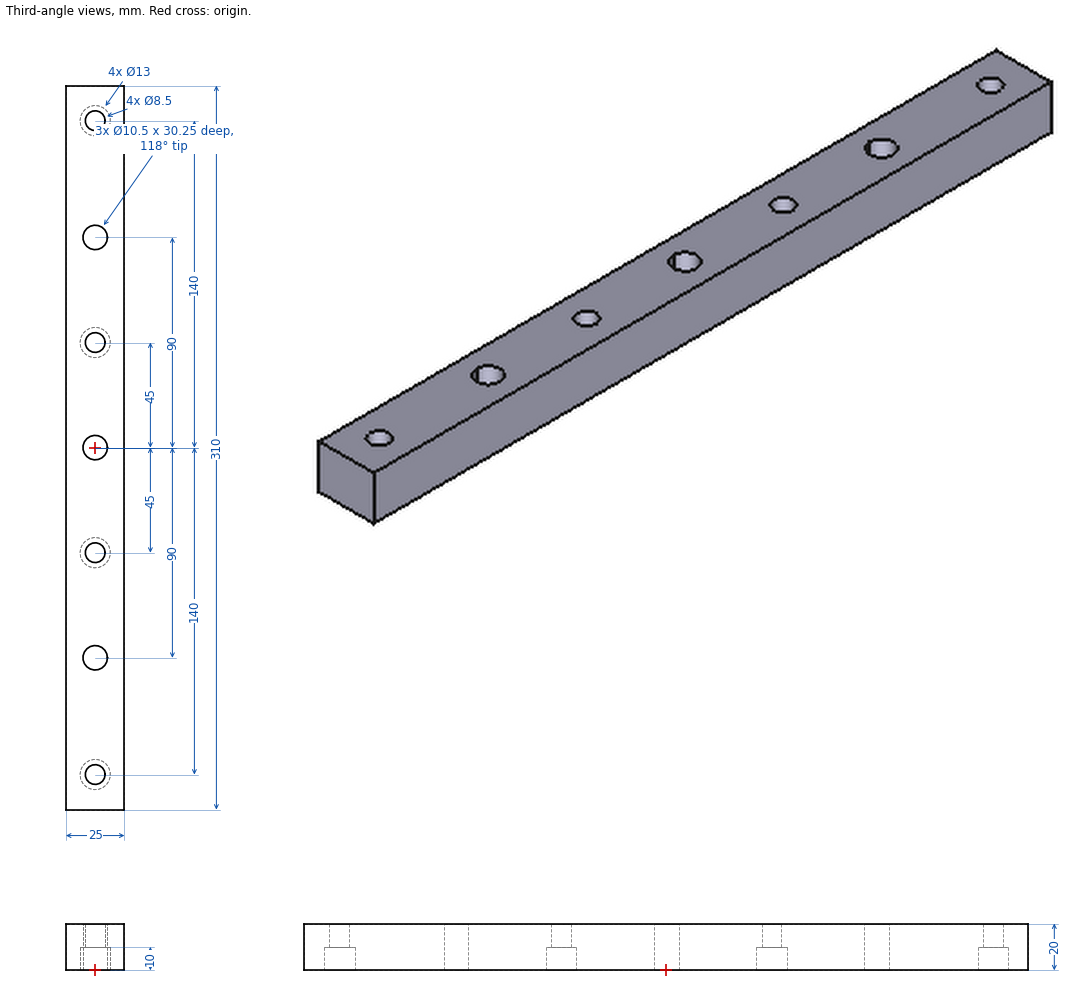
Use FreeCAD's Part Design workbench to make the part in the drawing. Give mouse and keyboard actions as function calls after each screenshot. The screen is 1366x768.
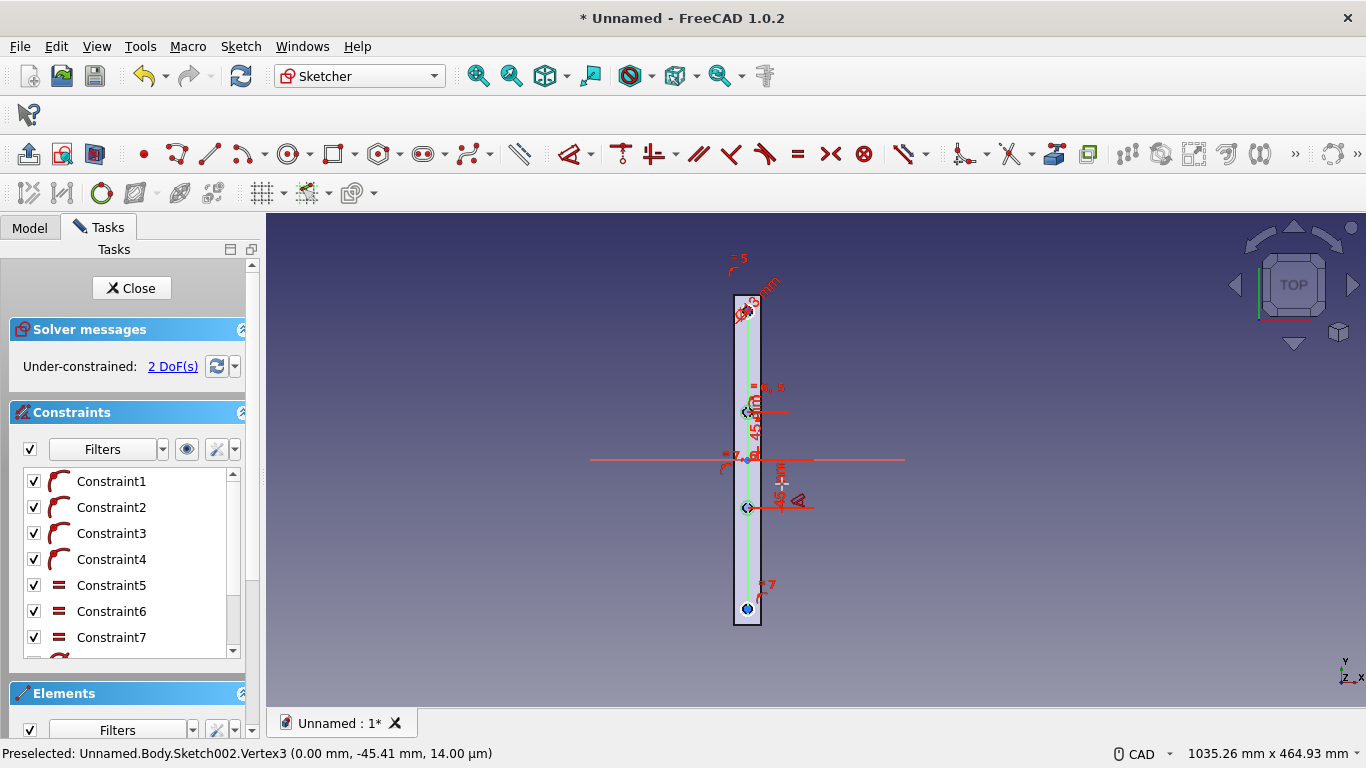
click(748, 312)
click(782, 386)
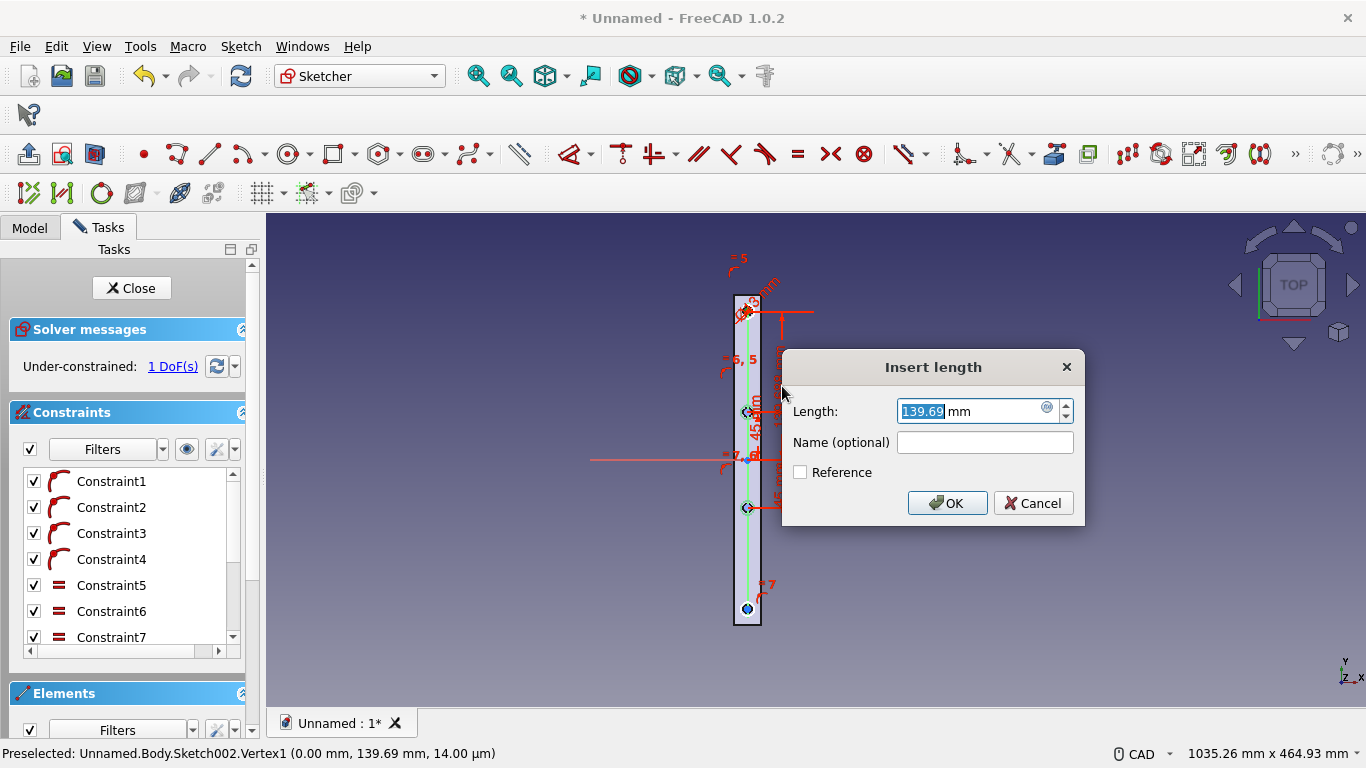
text(140)
key(Return)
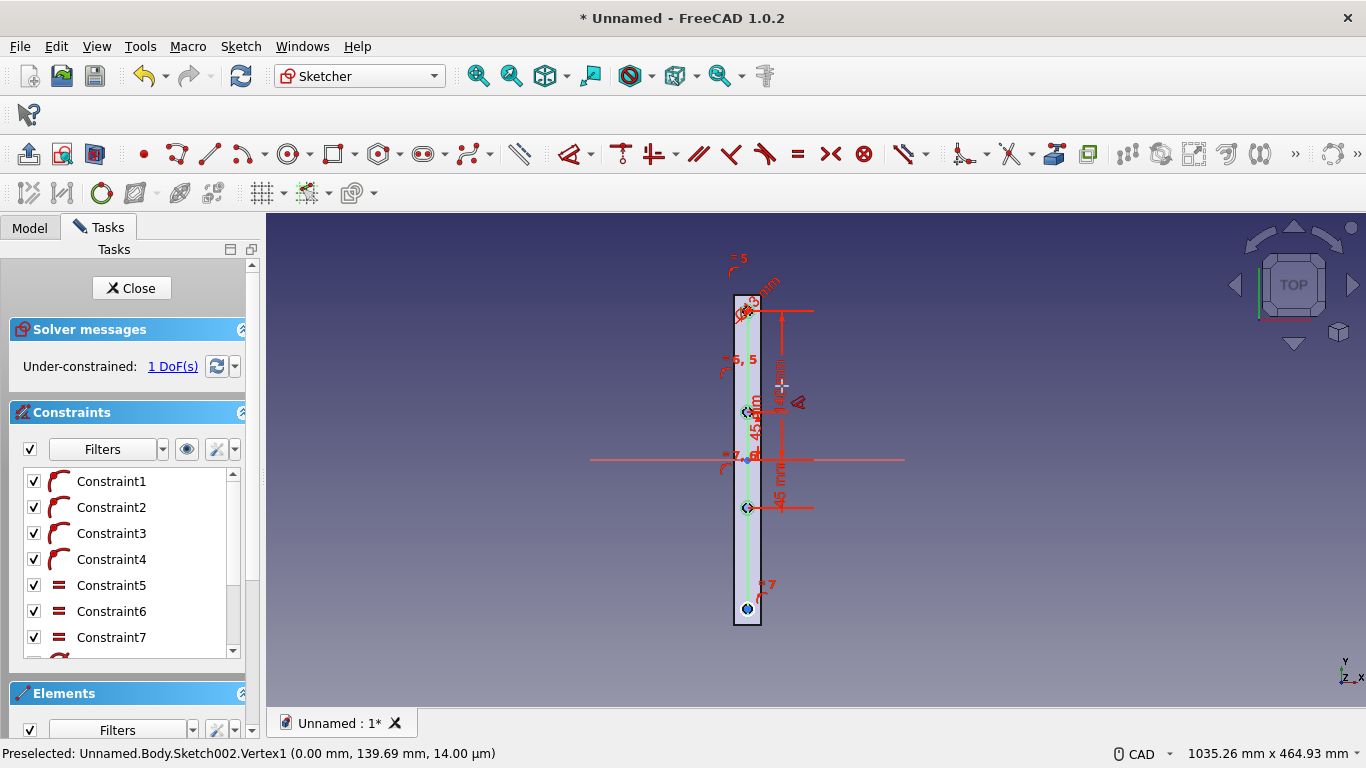
click(748, 609)
click(782, 535)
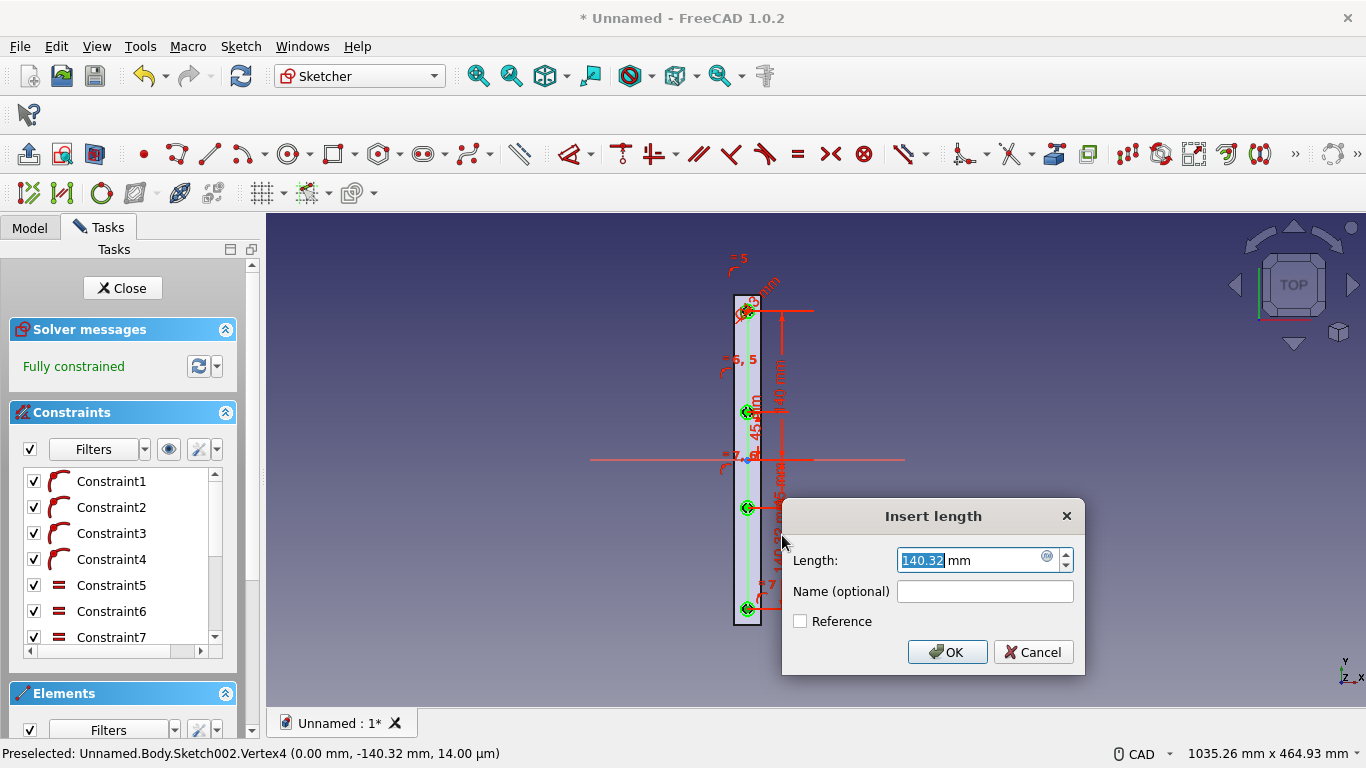
text(140)
key(Return)
key(Escape)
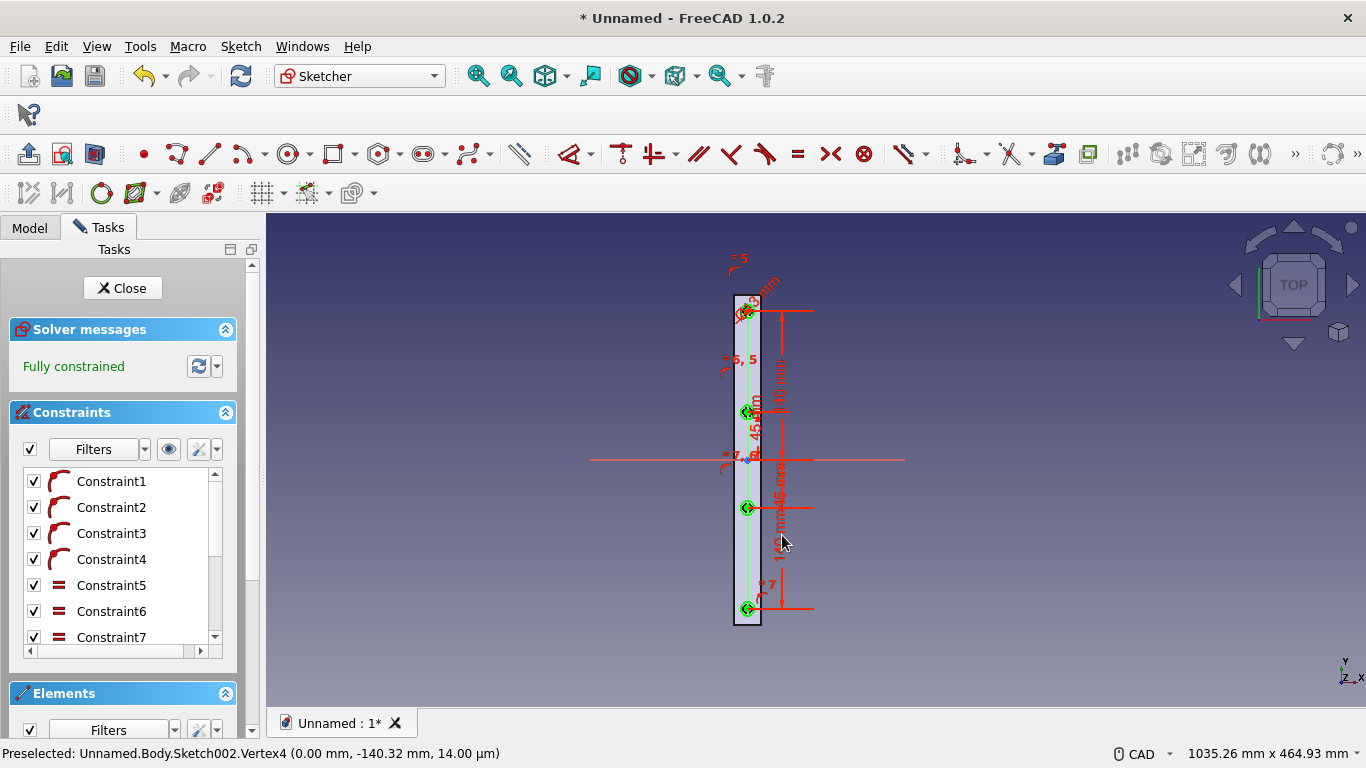
click(123, 288)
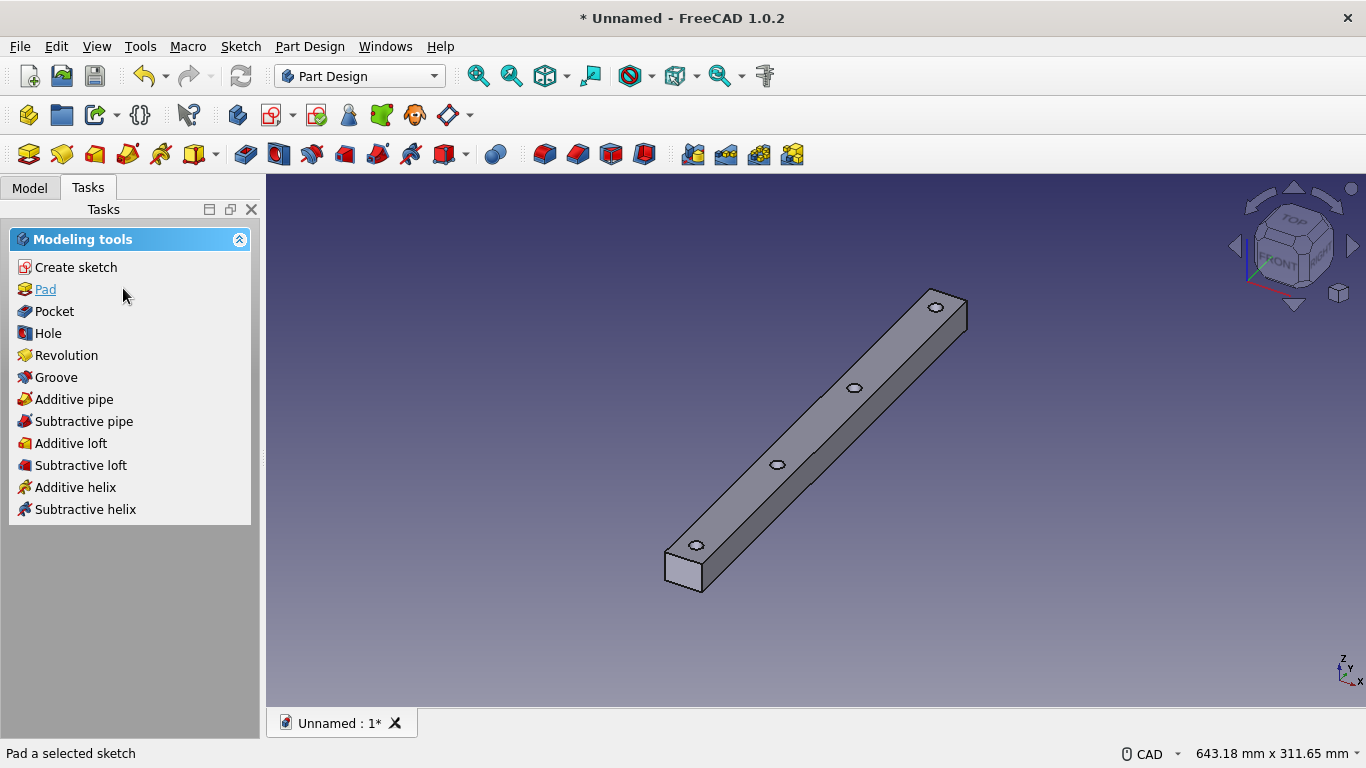
click(246, 154)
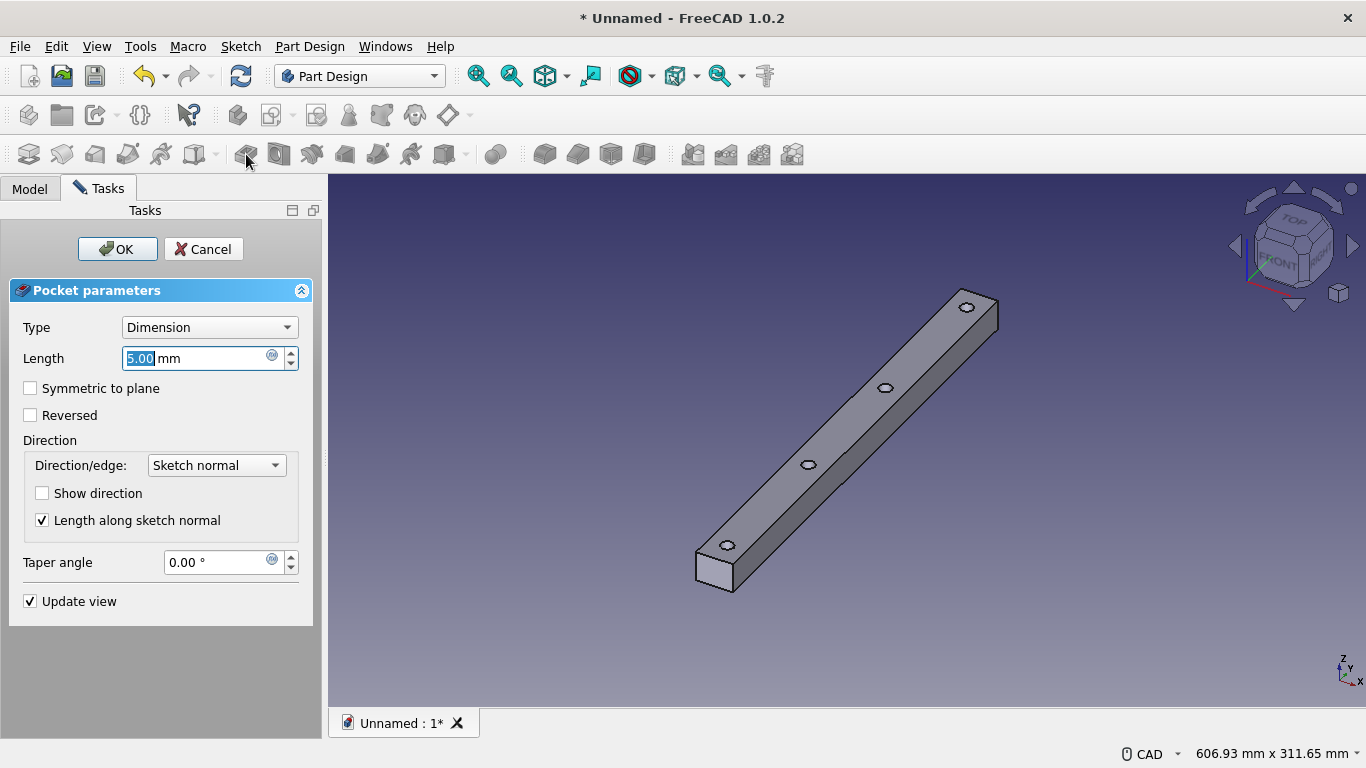
text(10)
key(Tab)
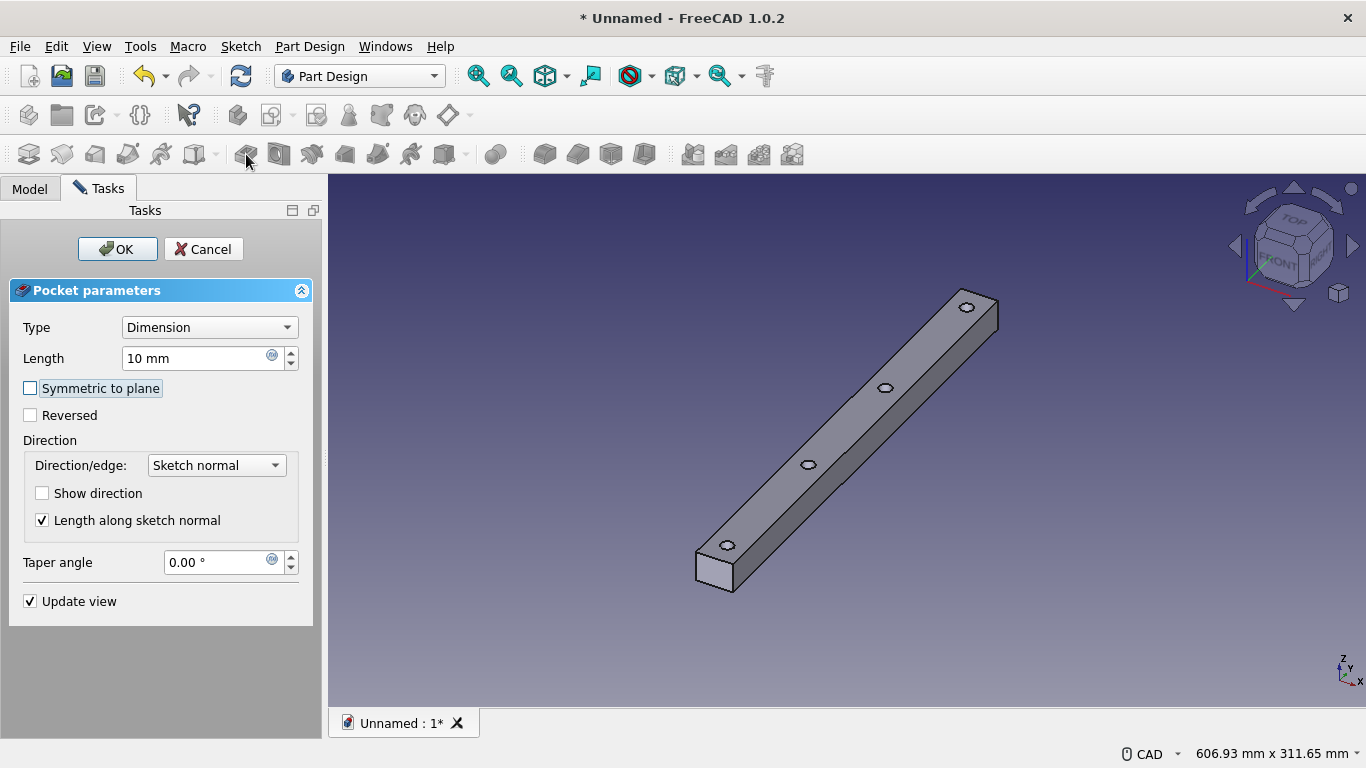
click(31, 415)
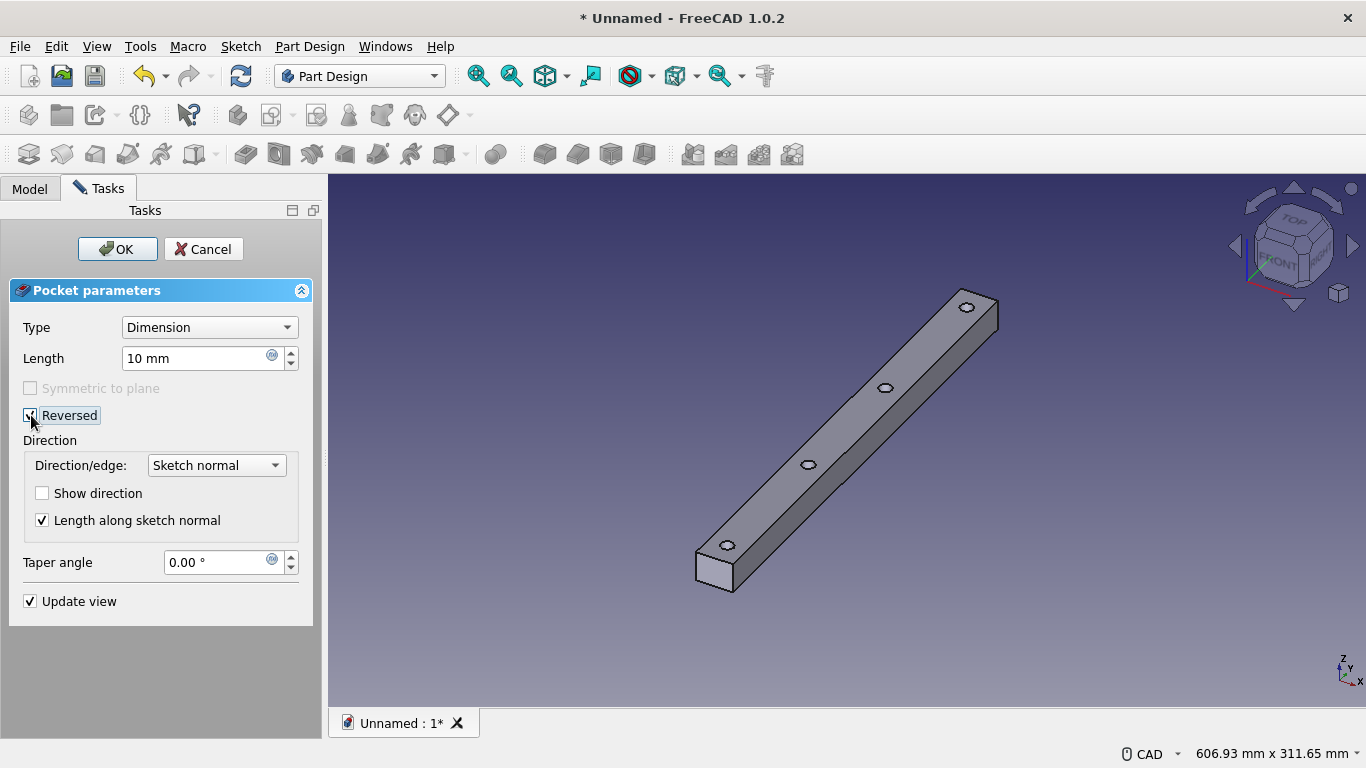
click(118, 249)